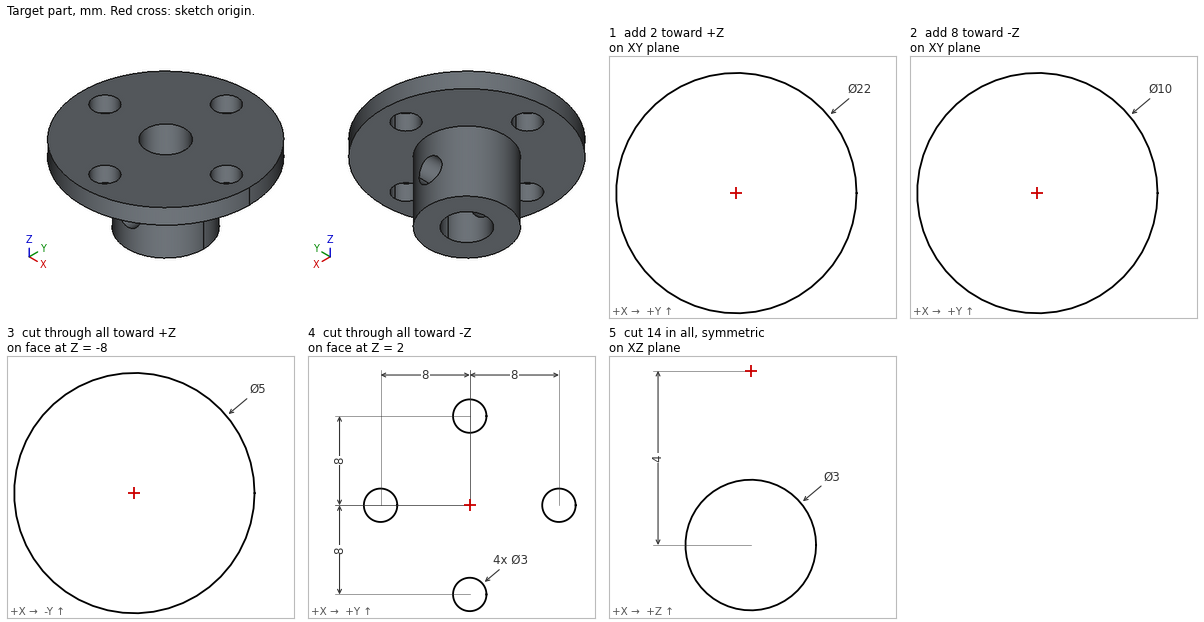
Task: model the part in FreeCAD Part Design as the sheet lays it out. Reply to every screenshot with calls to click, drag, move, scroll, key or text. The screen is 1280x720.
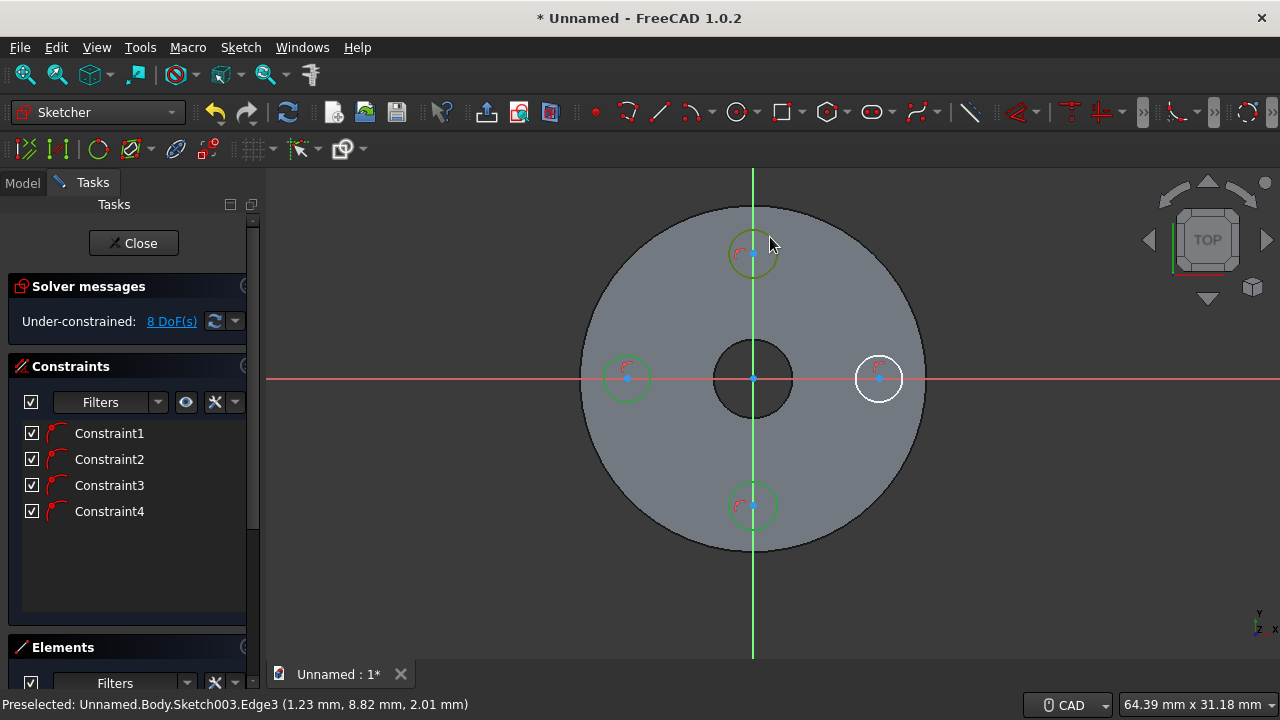
click(895, 362)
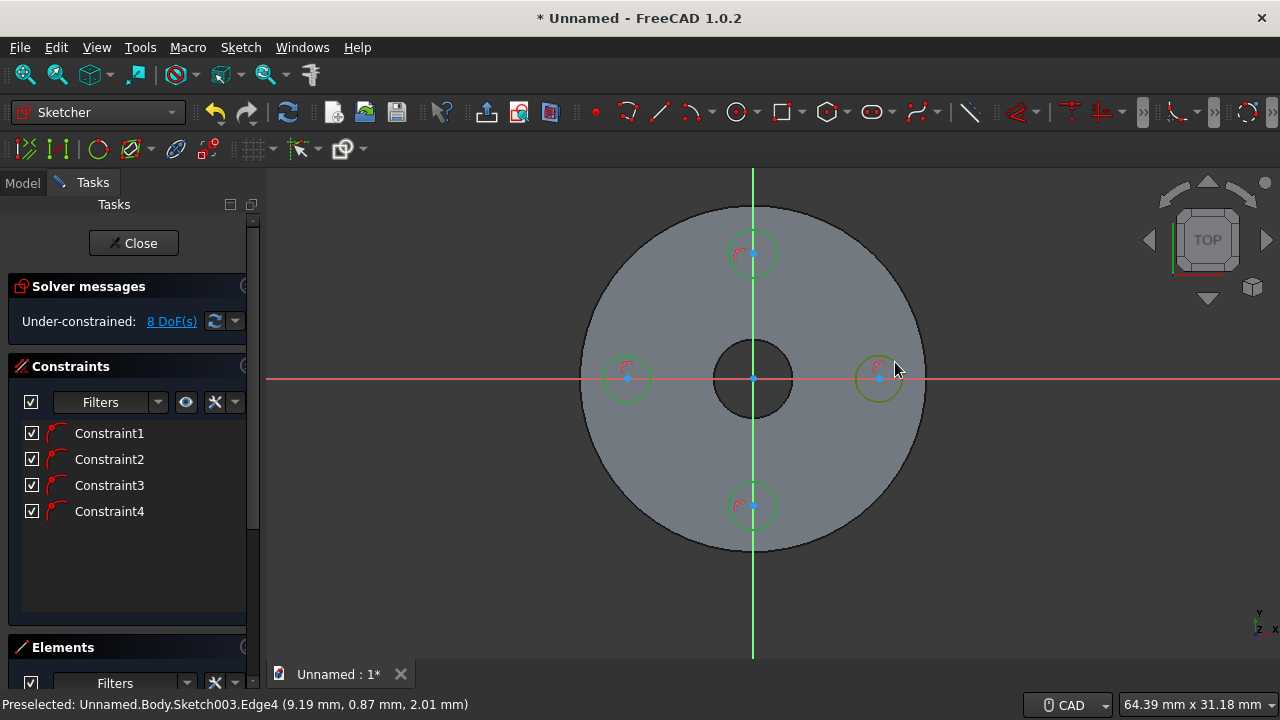
key(e)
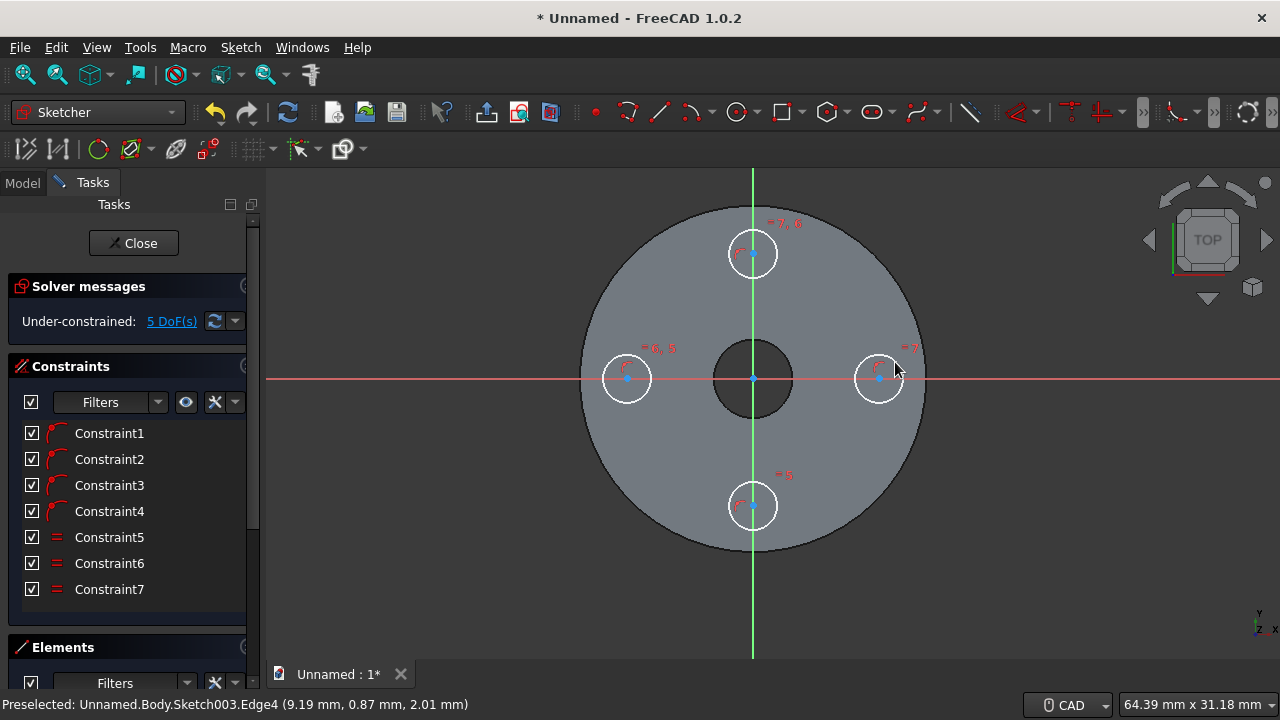
click(770, 489)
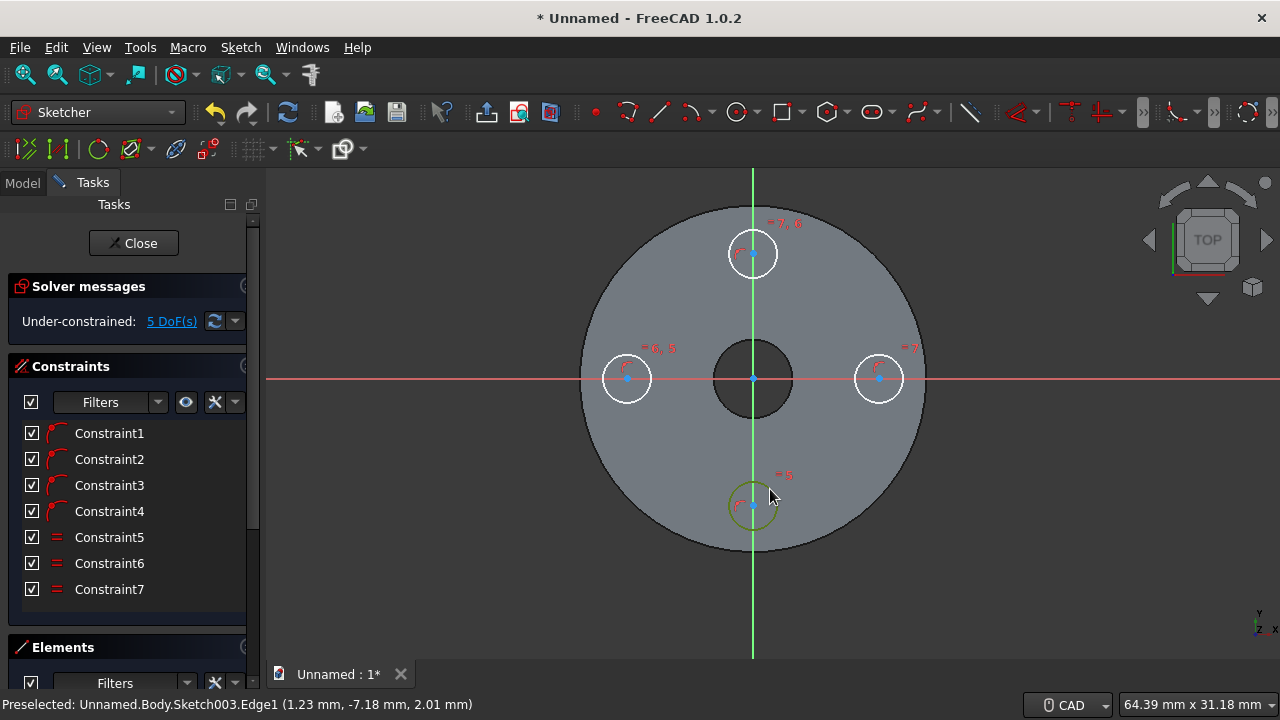
key(k)
key(o)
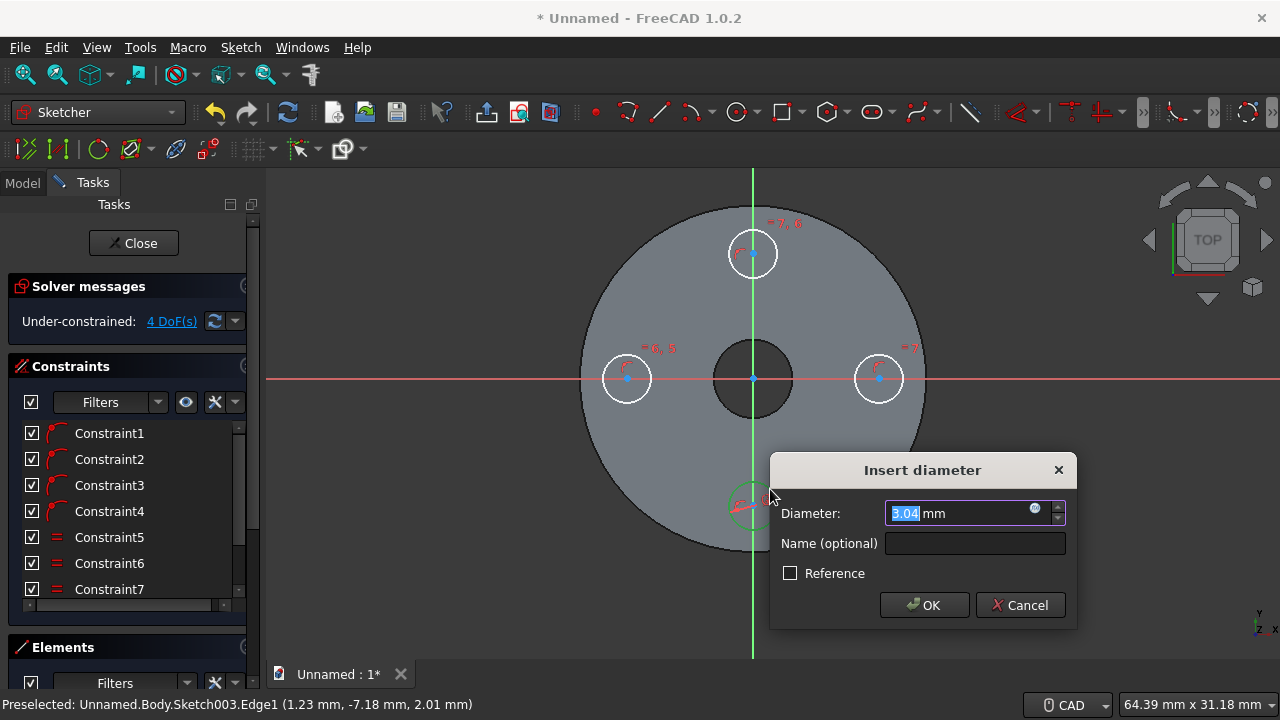
text(3)
key(Return)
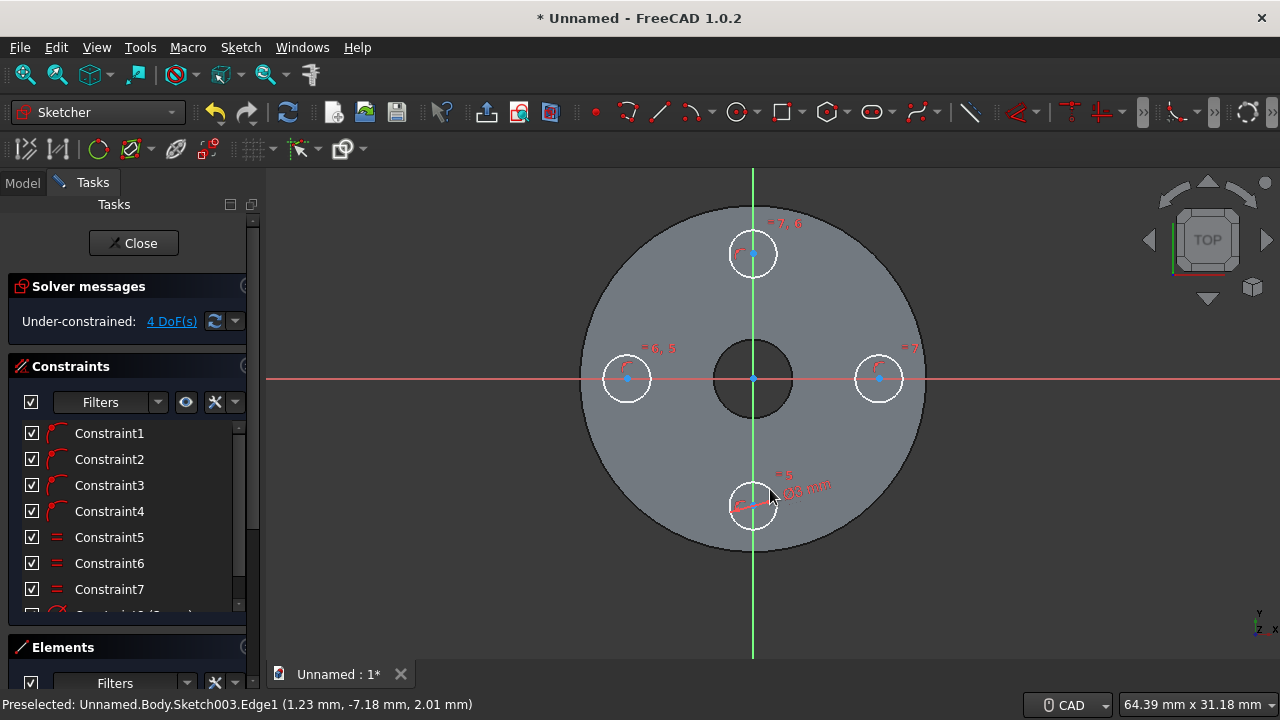
click(753, 506)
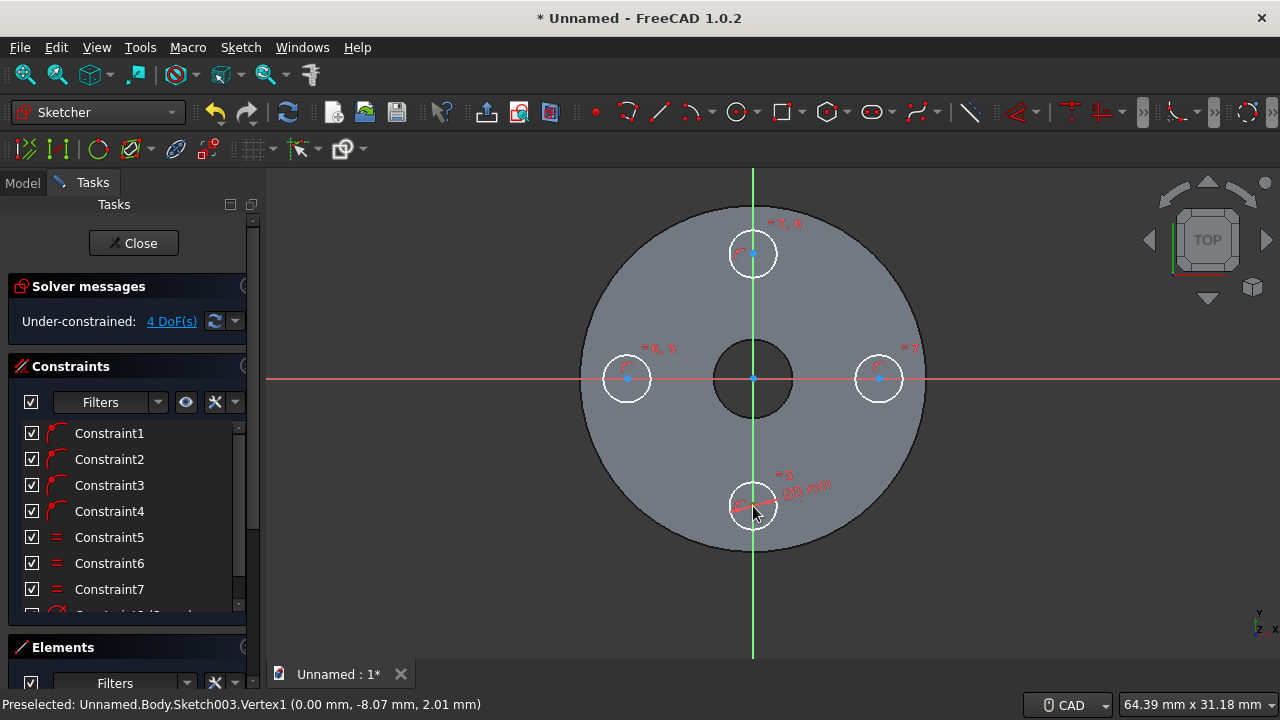
key(i)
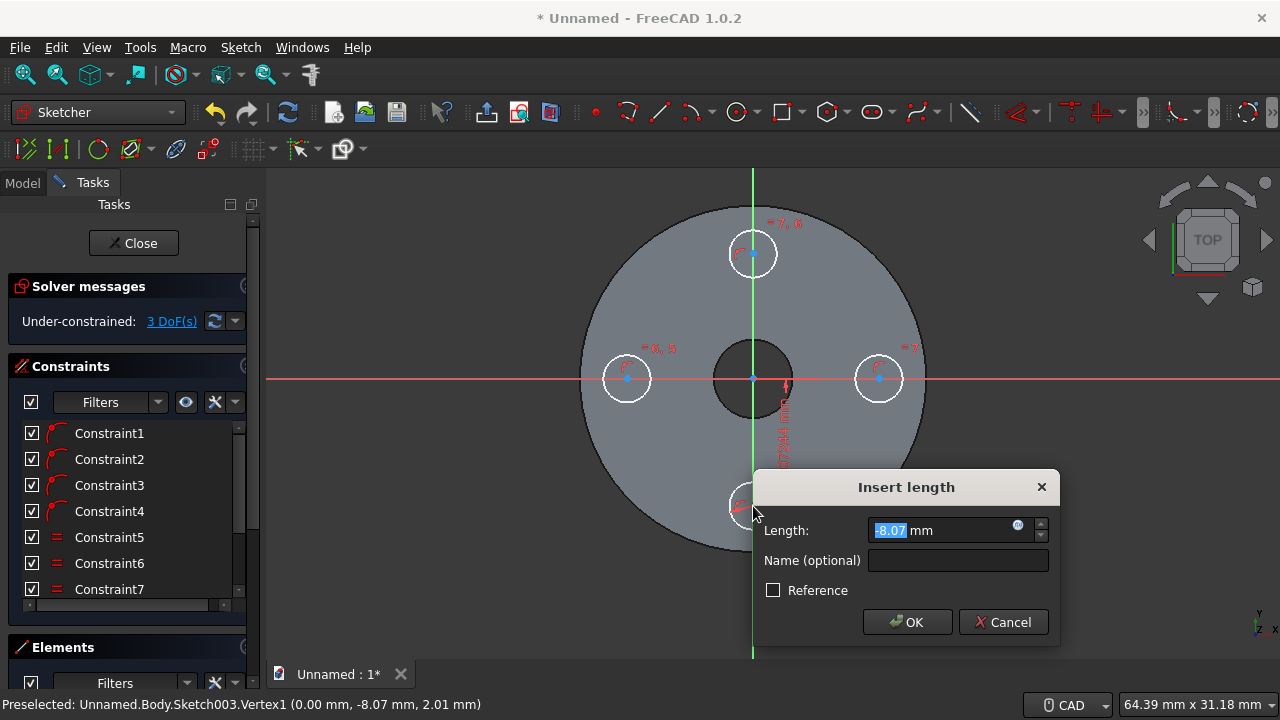
text(-8)
key(Return)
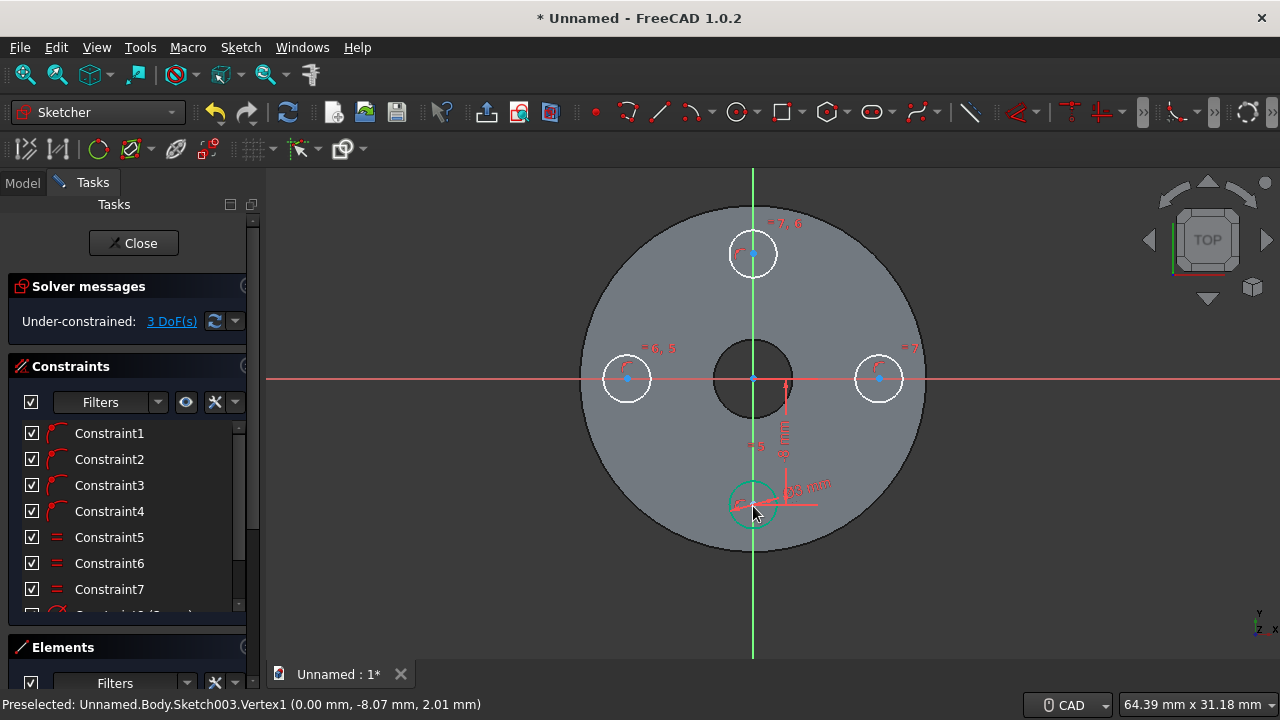
click(627, 379)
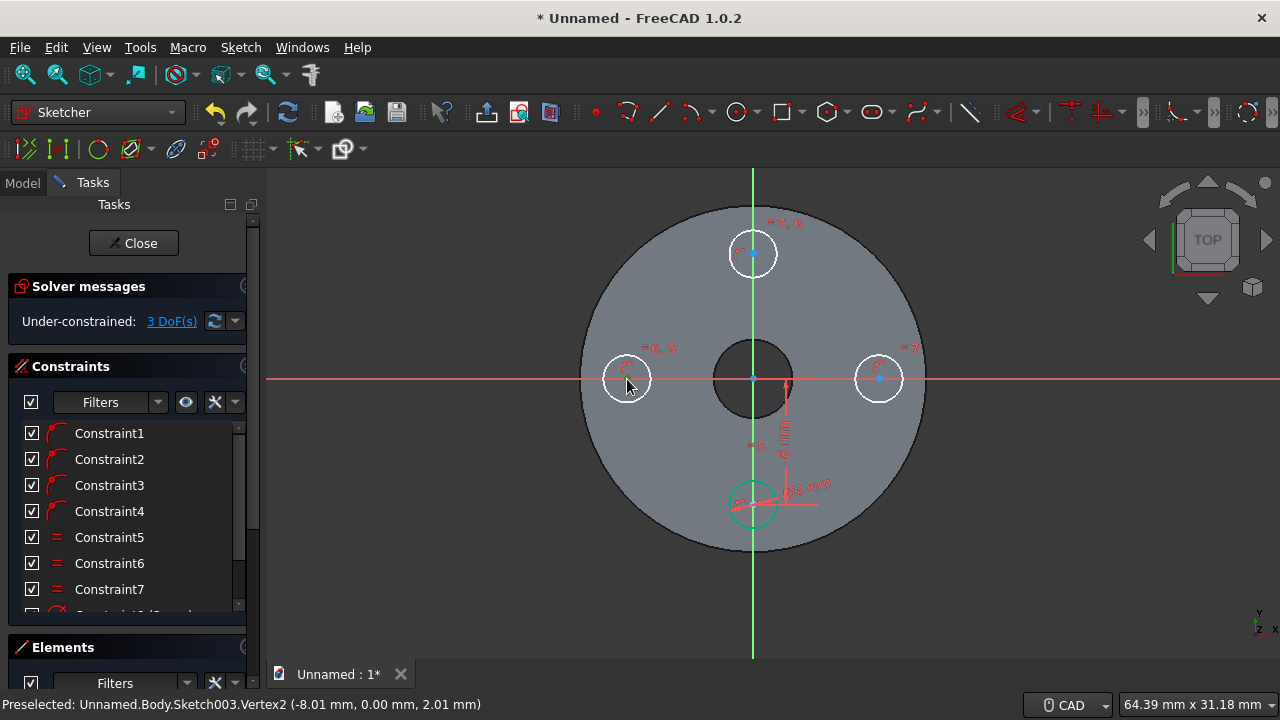
key(l)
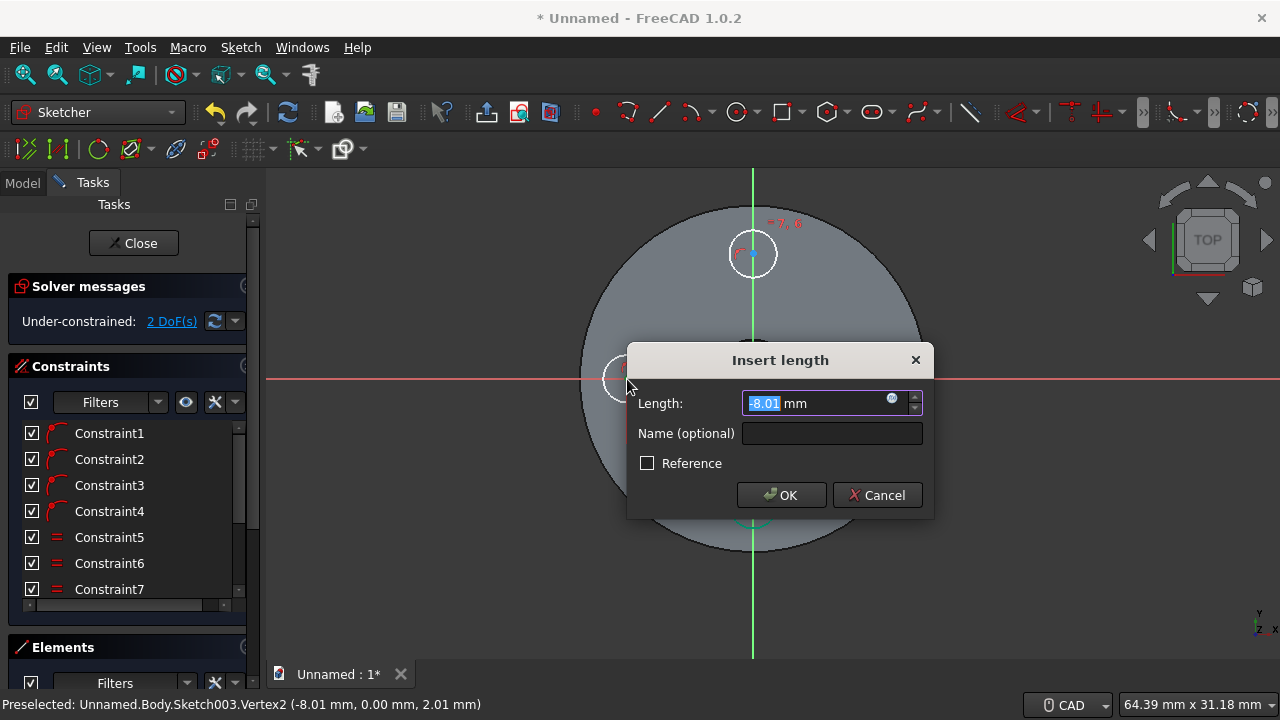
text(-8)
key(Return)